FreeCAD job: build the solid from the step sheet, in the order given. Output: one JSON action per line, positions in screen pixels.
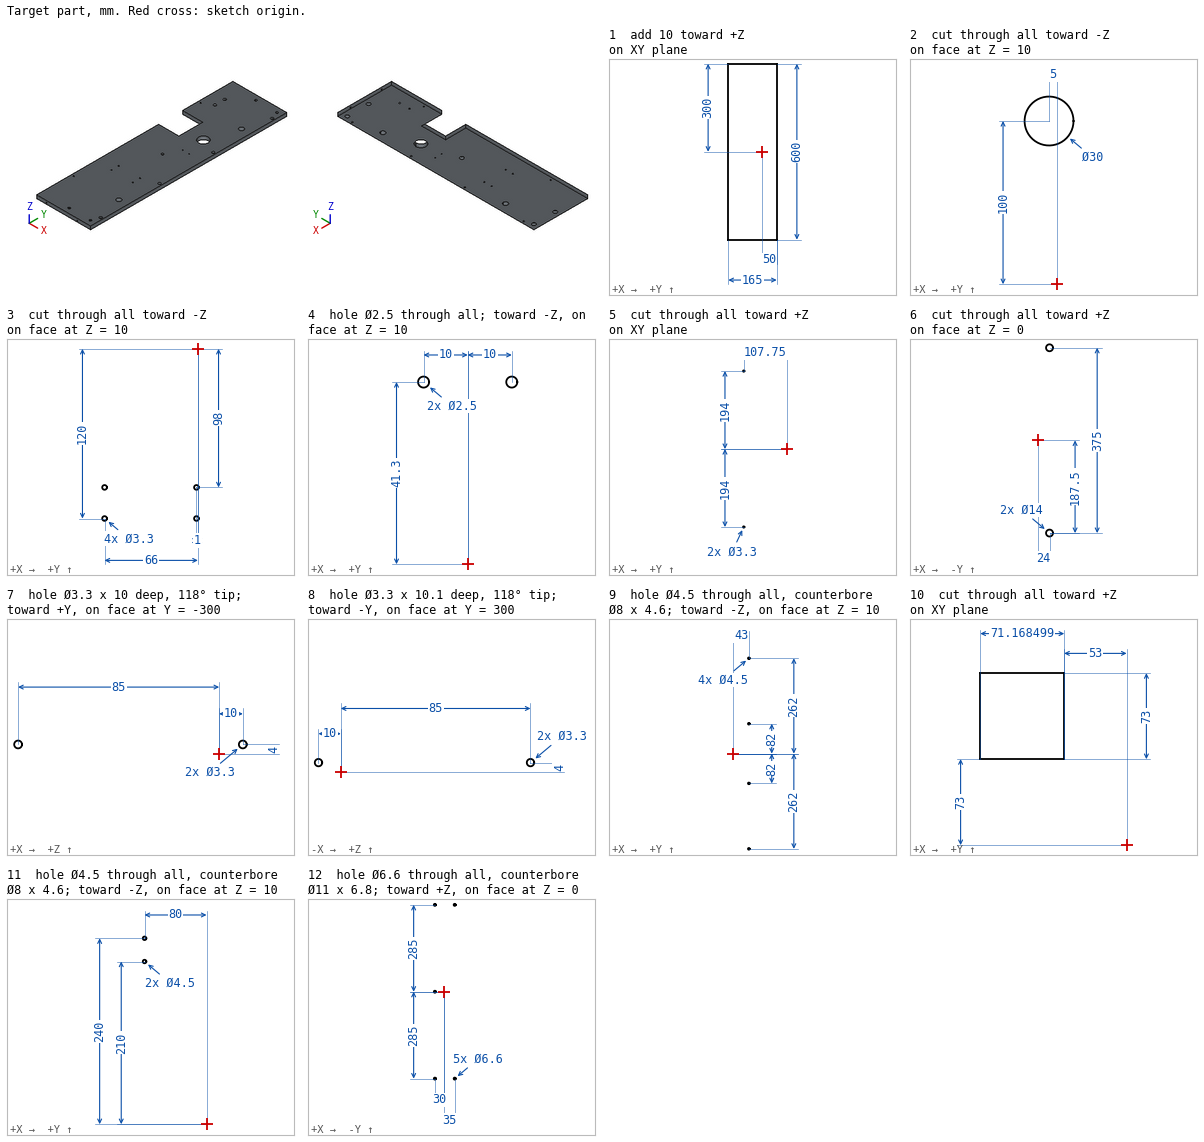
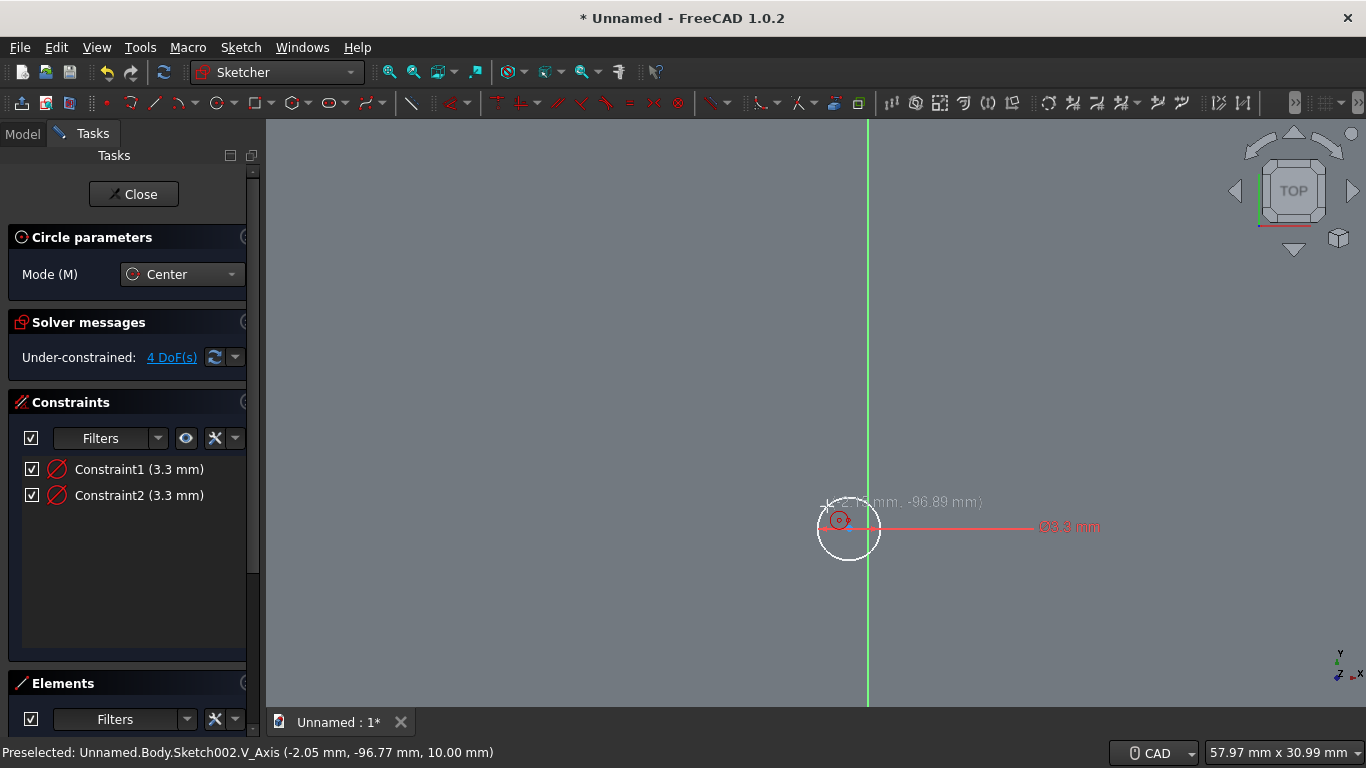
{"action": "scroll", "coordinate": [850, 530], "scroll_direction": "down", "scroll_amount": 9}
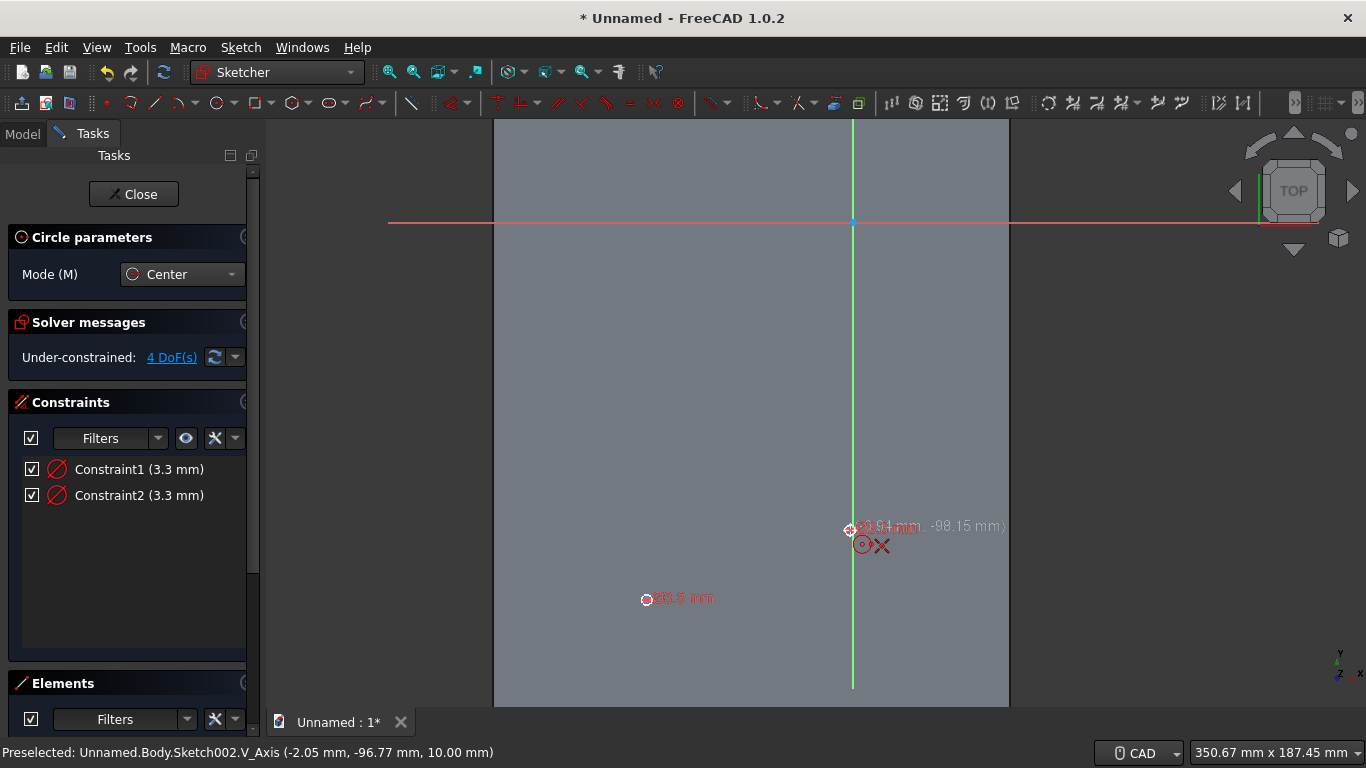
{"action": "scroll", "coordinate": [850, 599], "scroll_direction": "up", "scroll_amount": 9}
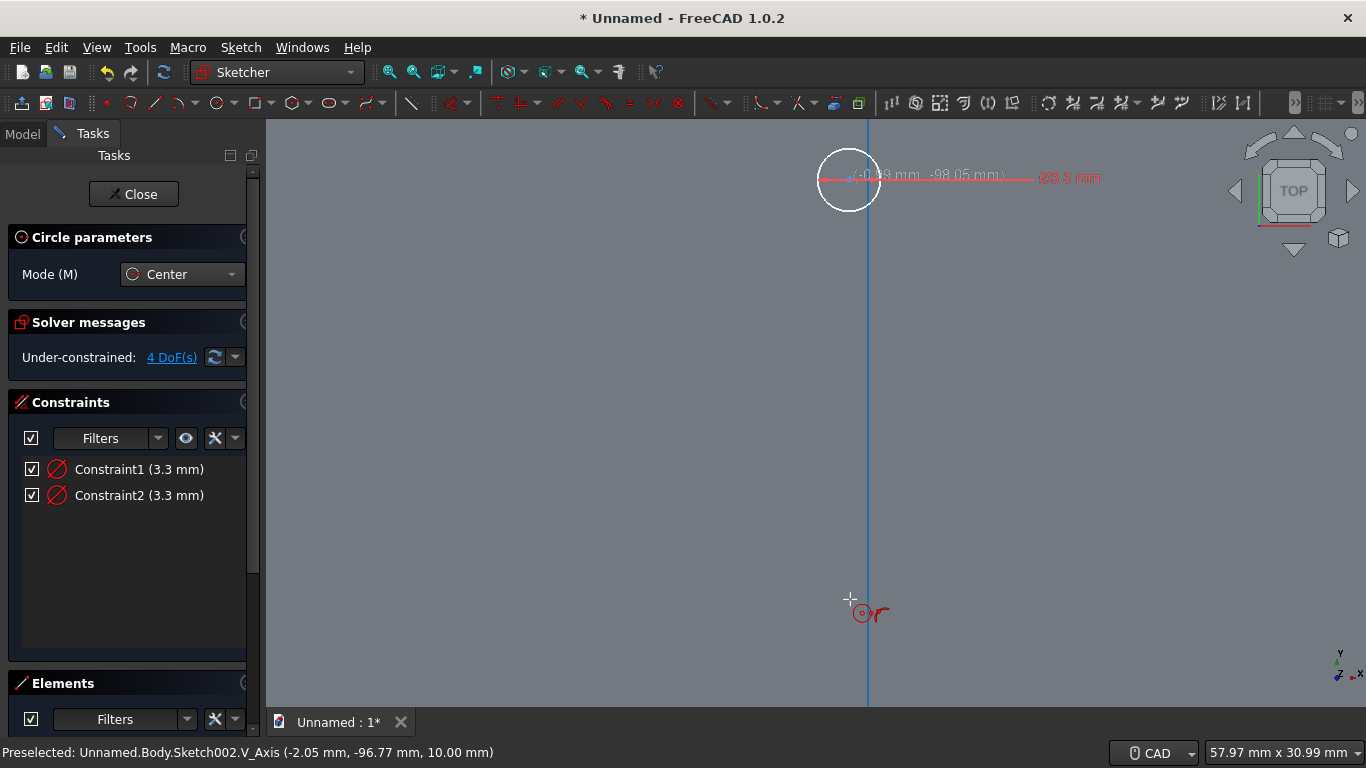
{"action": "left_click", "coordinate": [849, 597]}
{"action": "mouse_move", "coordinate": [827, 574]}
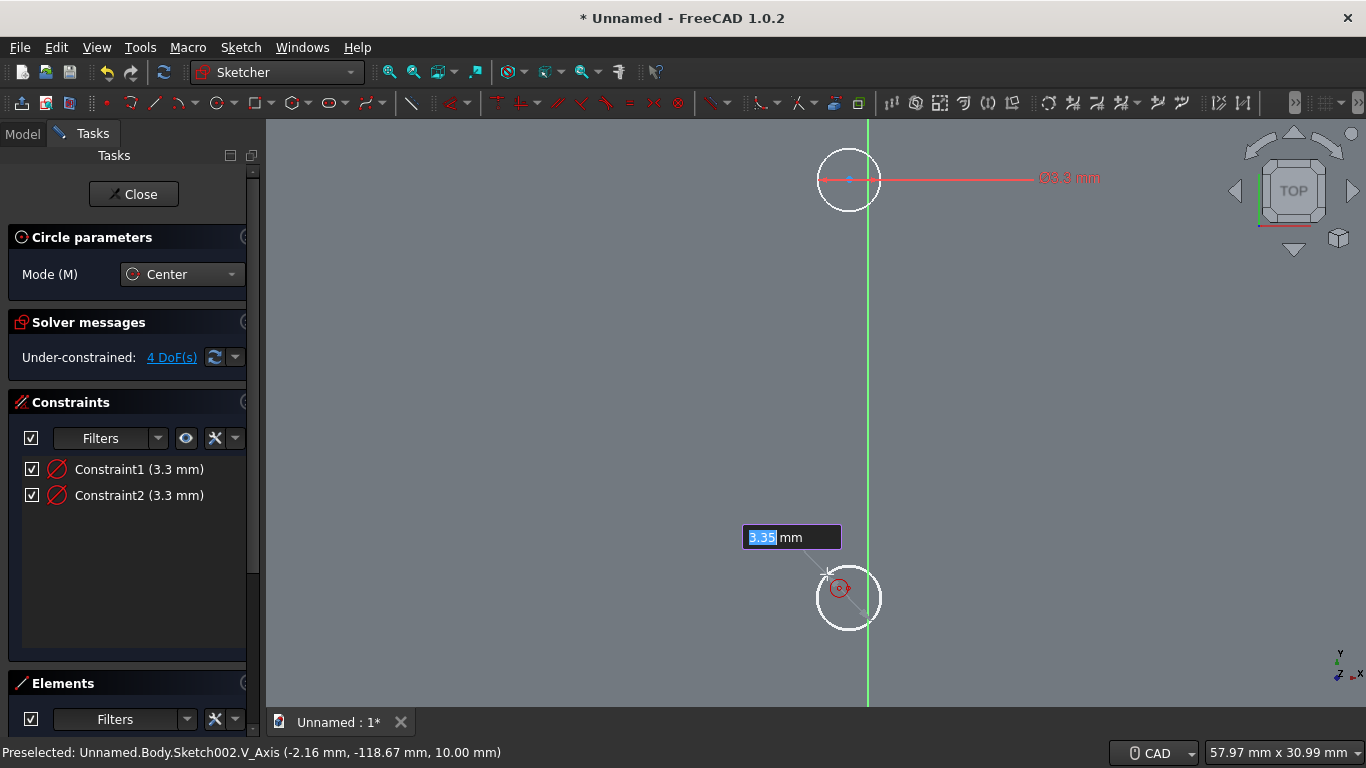
{"action": "type", "text": "3.3"}
{"action": "key", "text": "Return"}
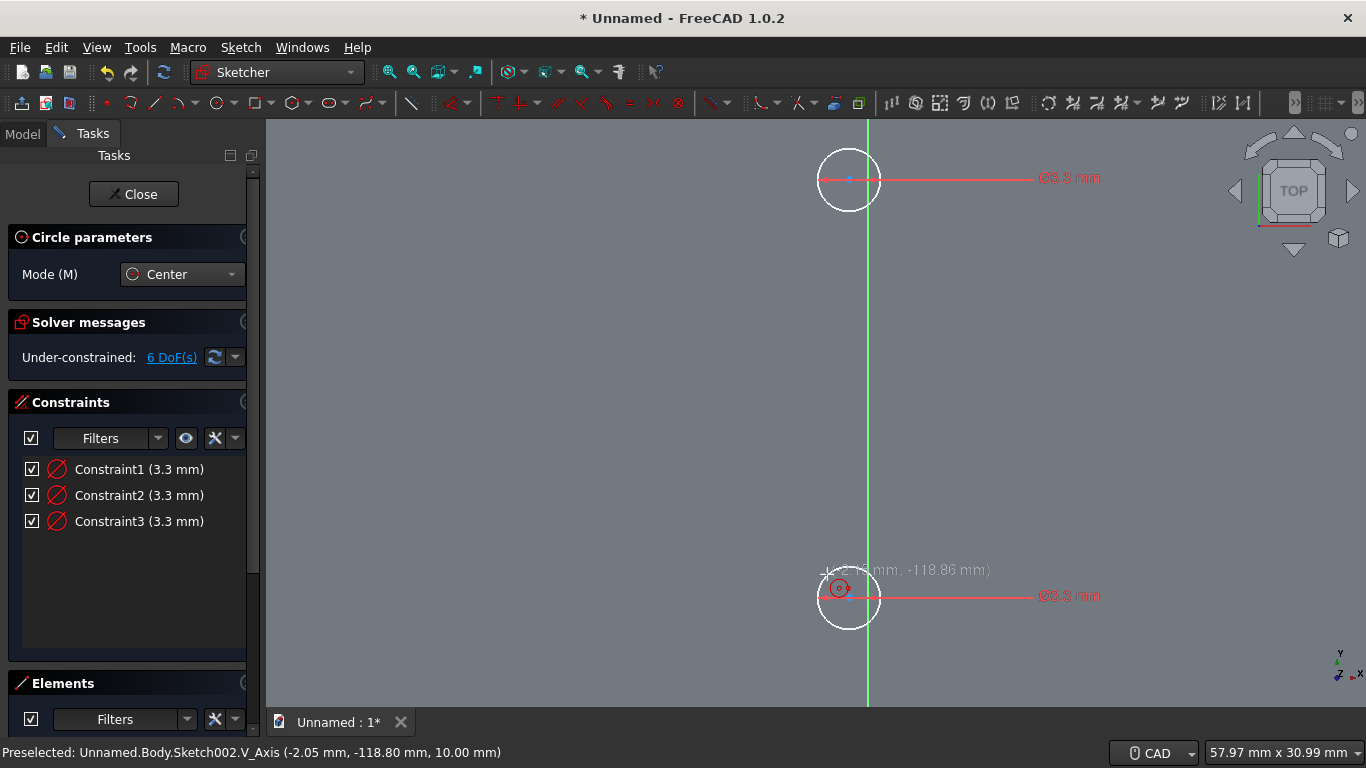
{"action": "scroll", "coordinate": [850, 599], "scroll_direction": "down", "scroll_amount": 9}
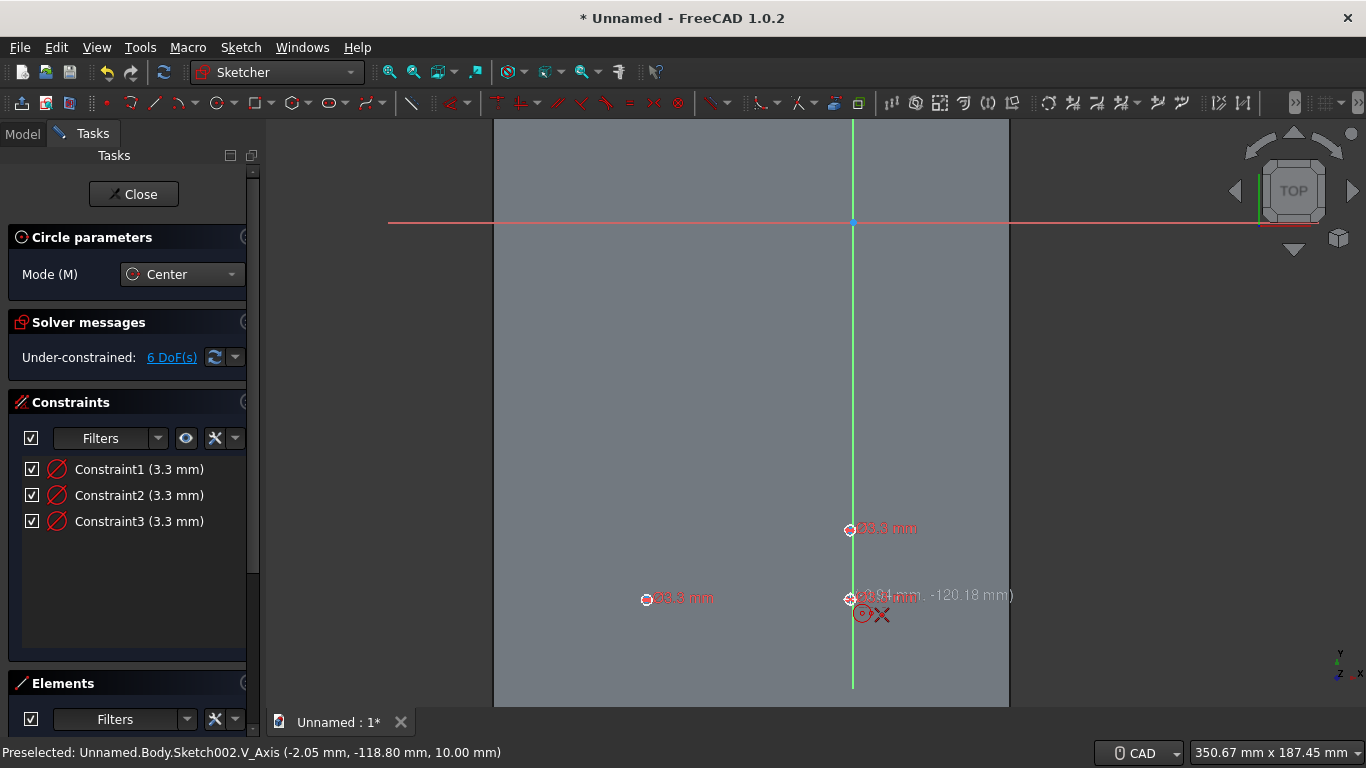
{"action": "scroll", "coordinate": [646, 530], "scroll_direction": "up", "scroll_amount": 8}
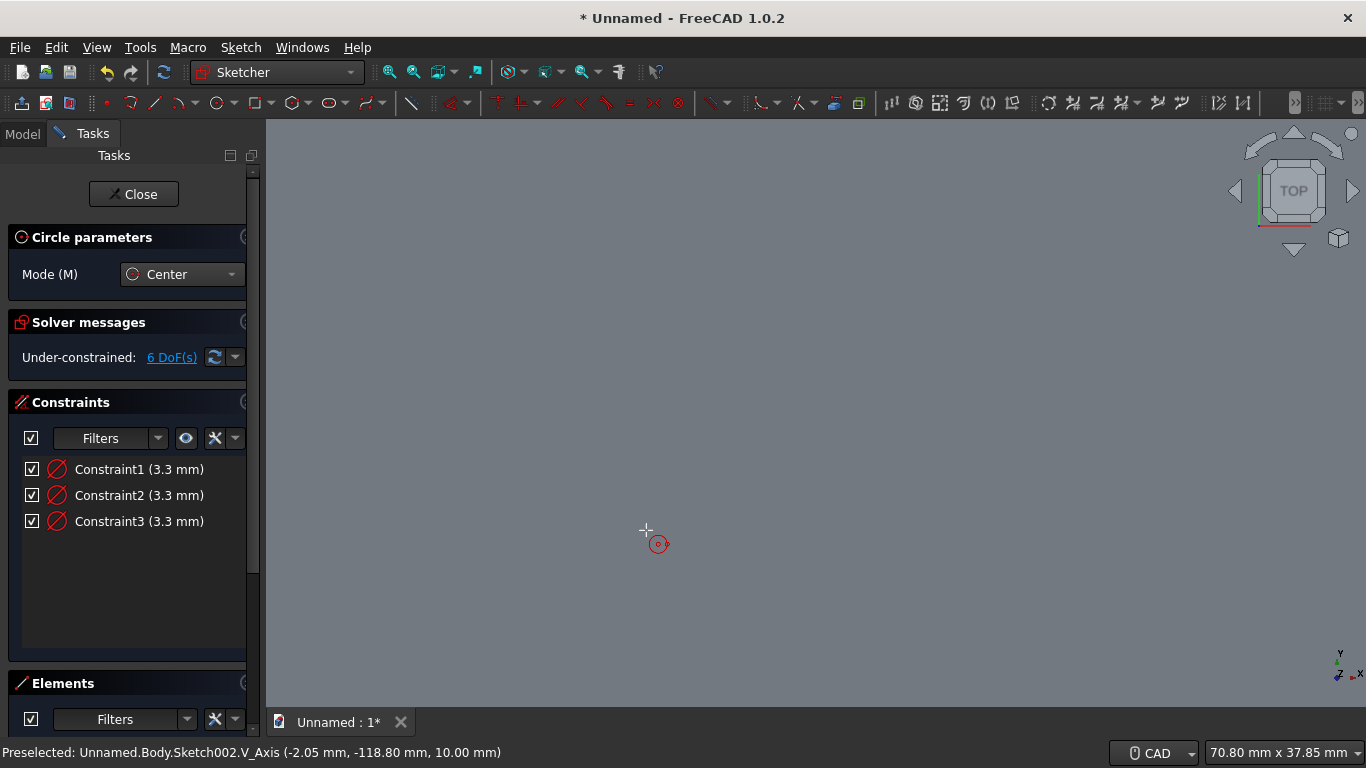
{"action": "scroll", "coordinate": [645, 530], "scroll_direction": "down", "scroll_amount": 8}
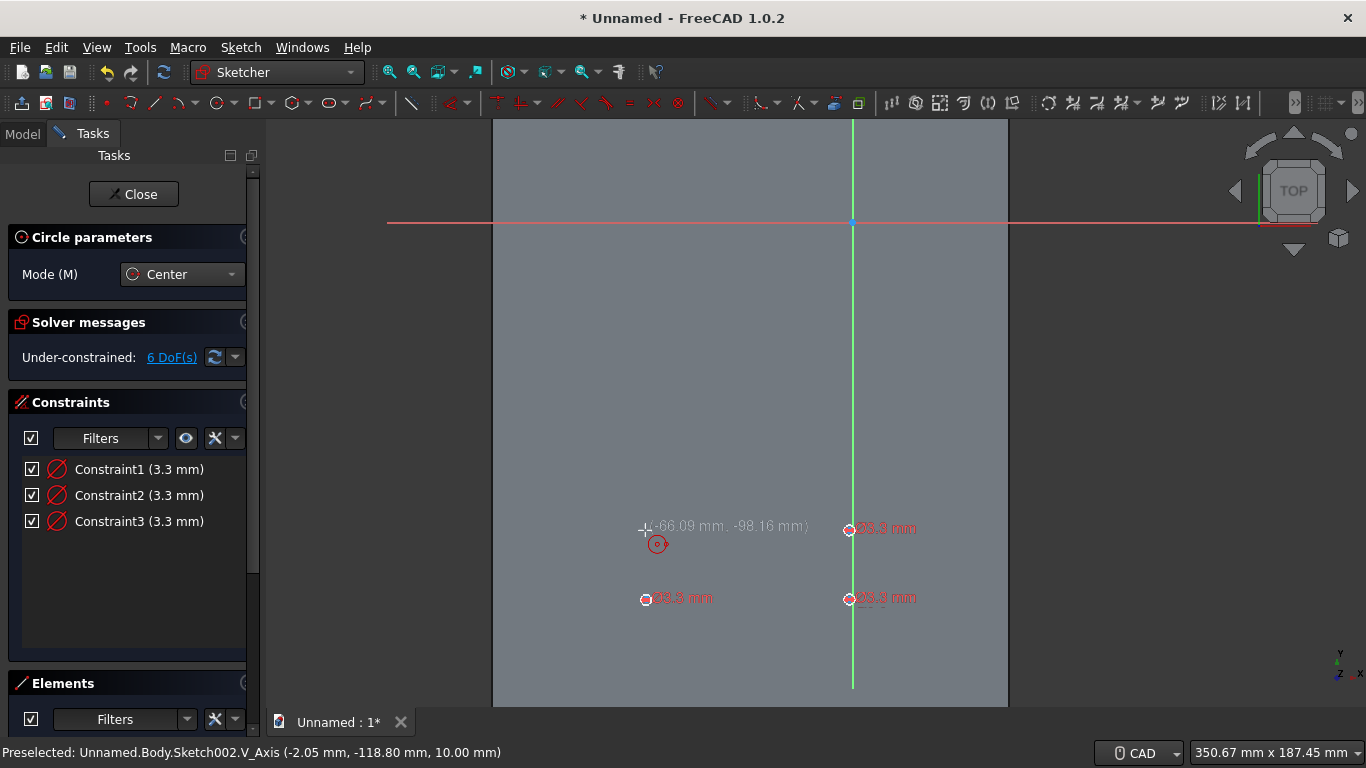
{"action": "left_click", "coordinate": [646, 530]}
{"action": "mouse_move", "coordinate": [649, 527]}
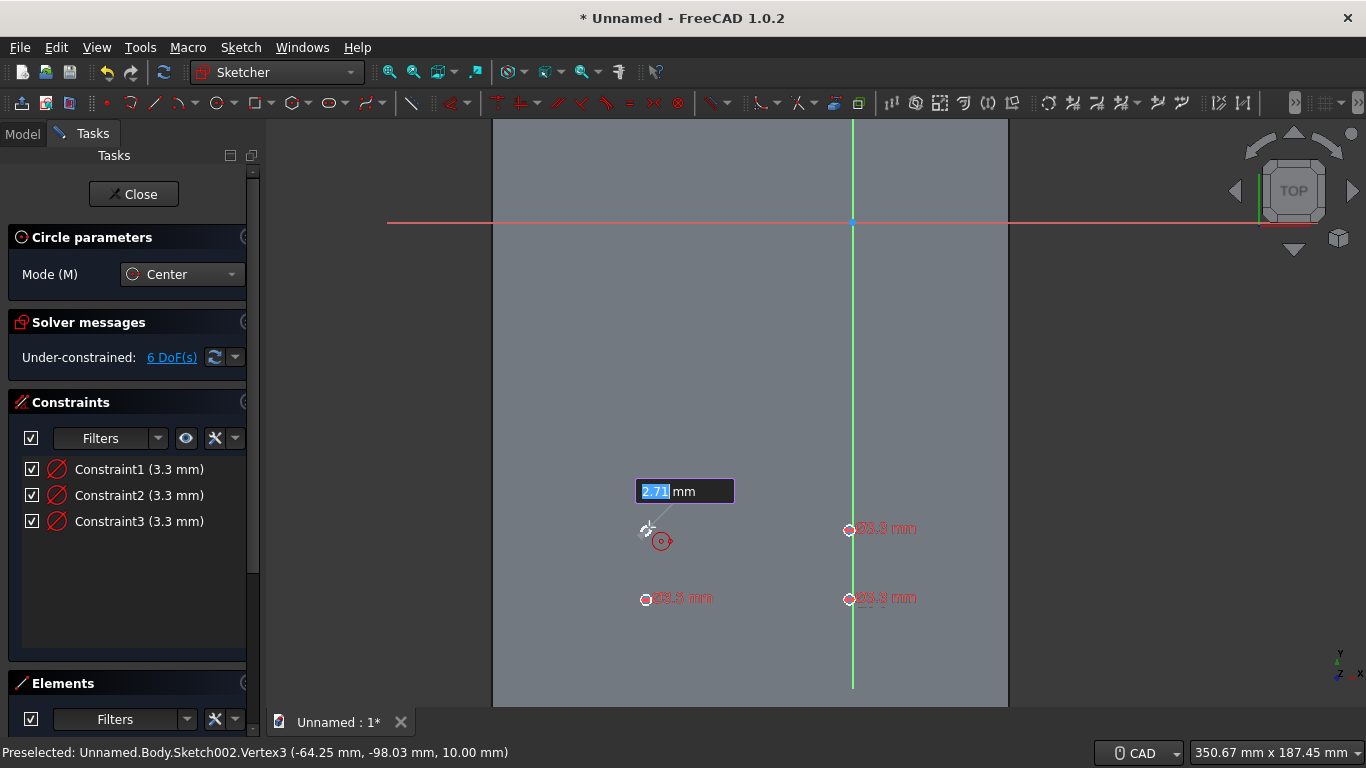
{"action": "type", "text": "3.3"}
{"action": "key", "text": "Return"}
{"action": "key", "text": "Escape"}